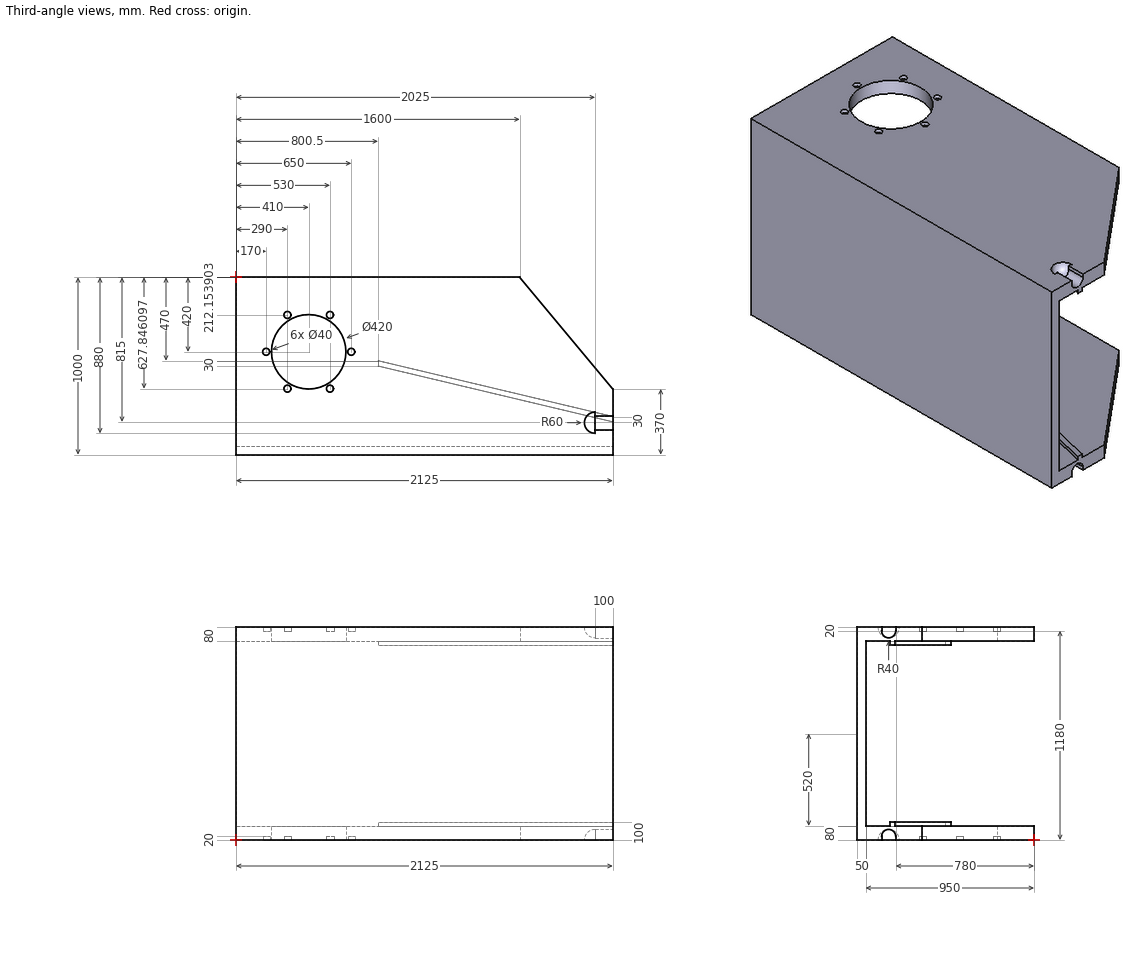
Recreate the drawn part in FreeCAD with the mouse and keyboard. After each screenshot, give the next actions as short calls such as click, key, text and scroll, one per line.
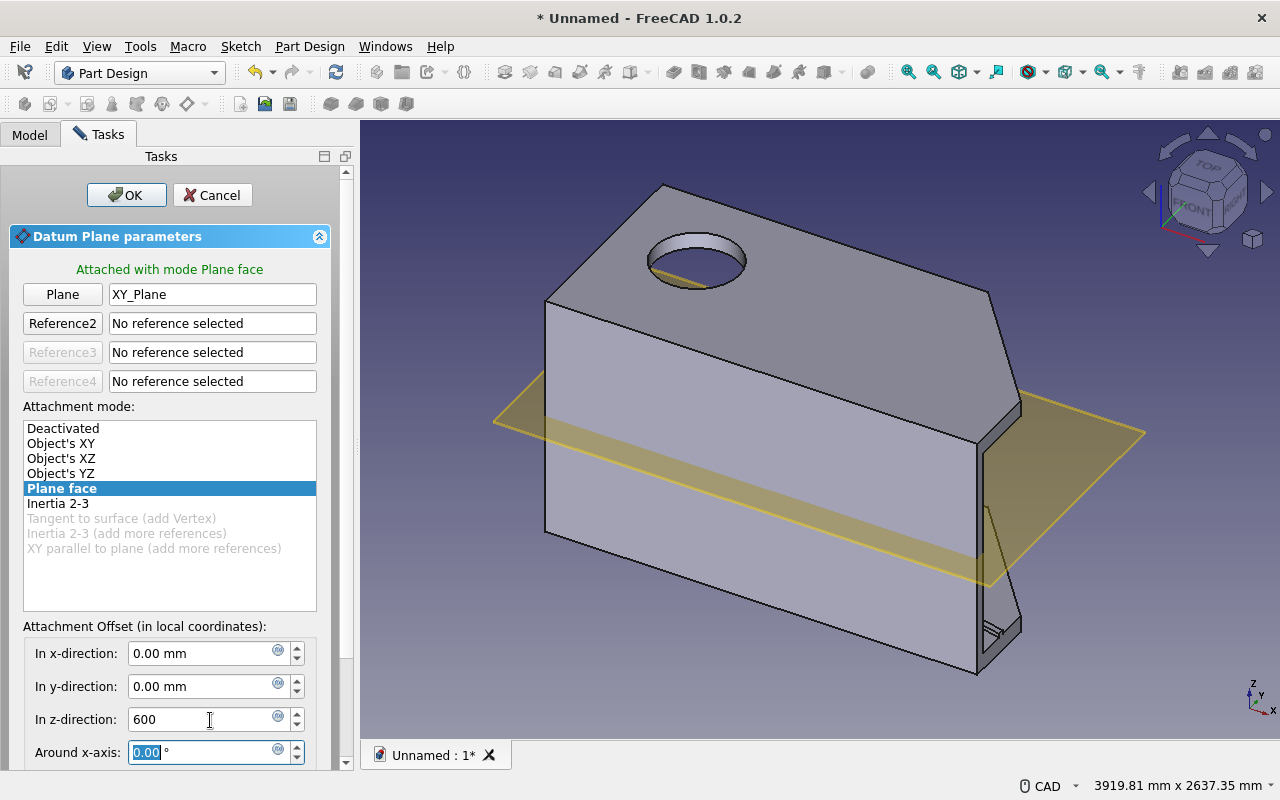
click(127, 195)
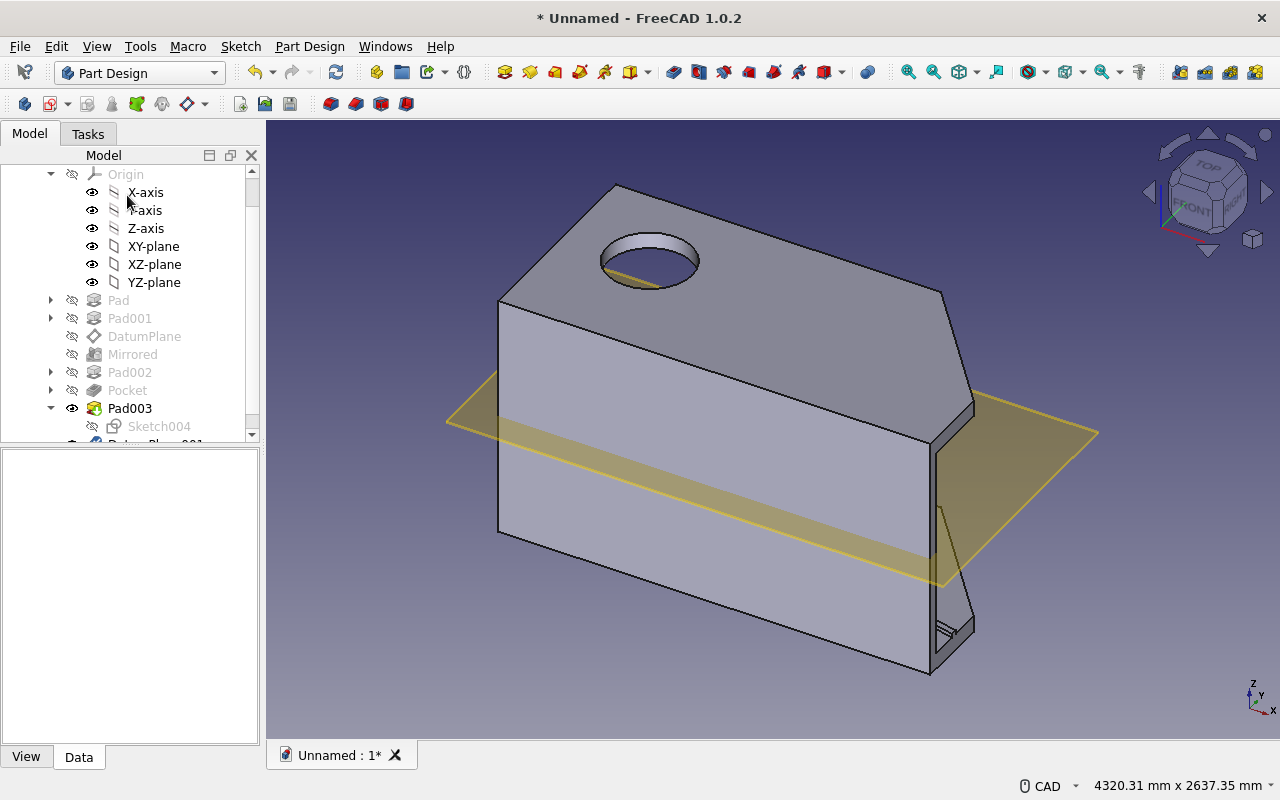
click(117, 408)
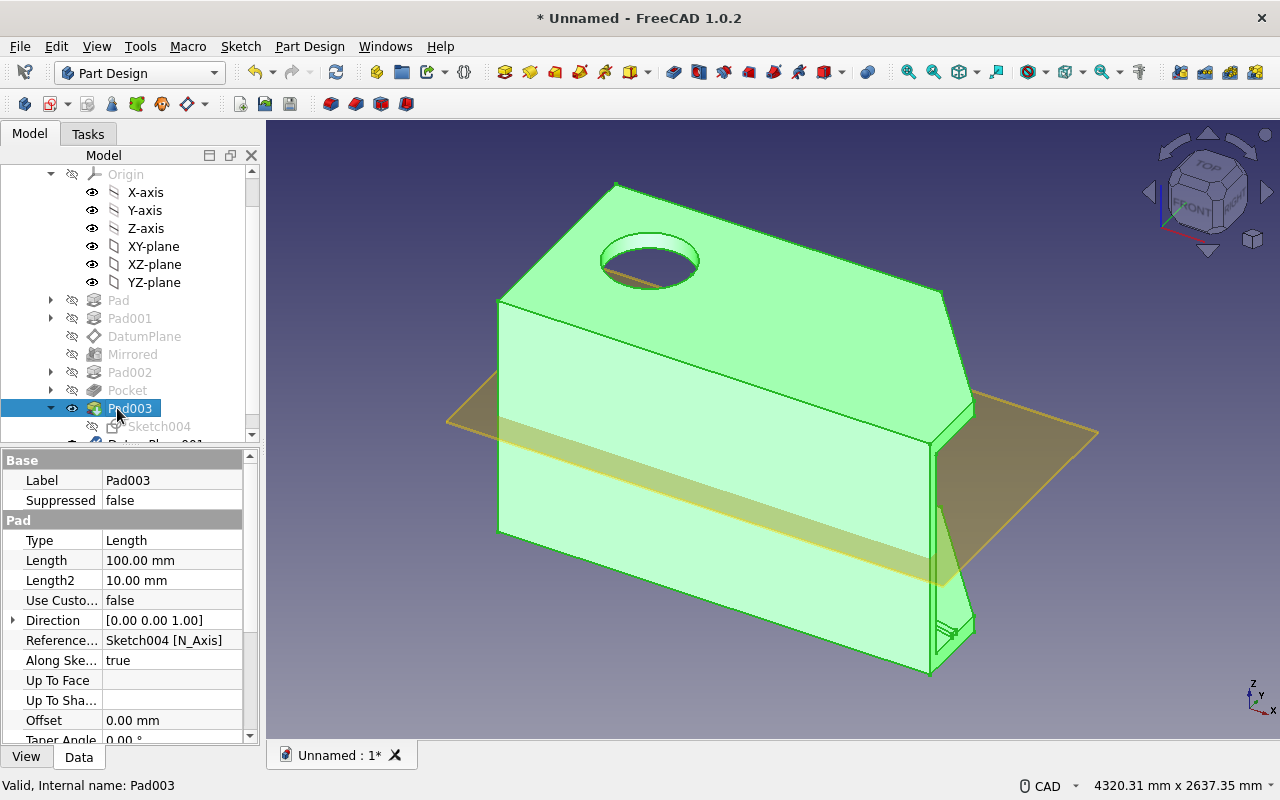
click(1180, 72)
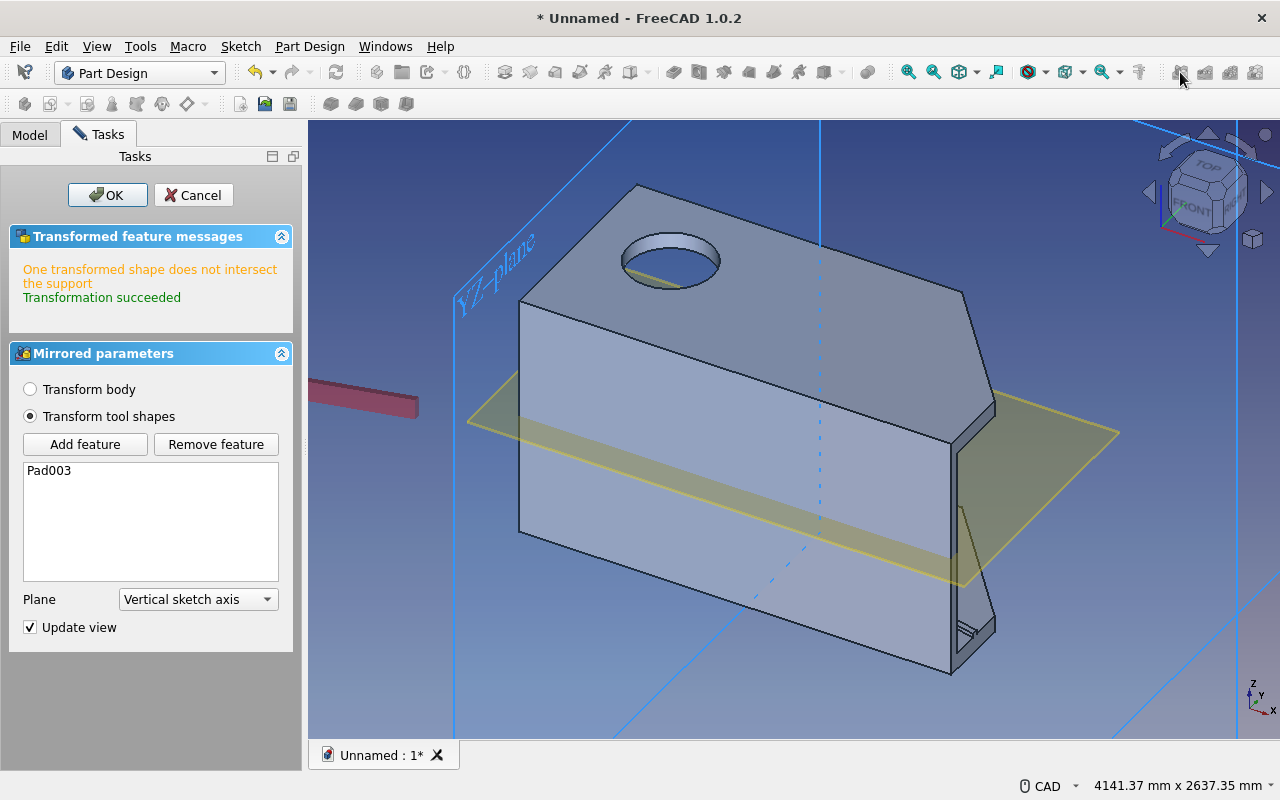
click(199, 600)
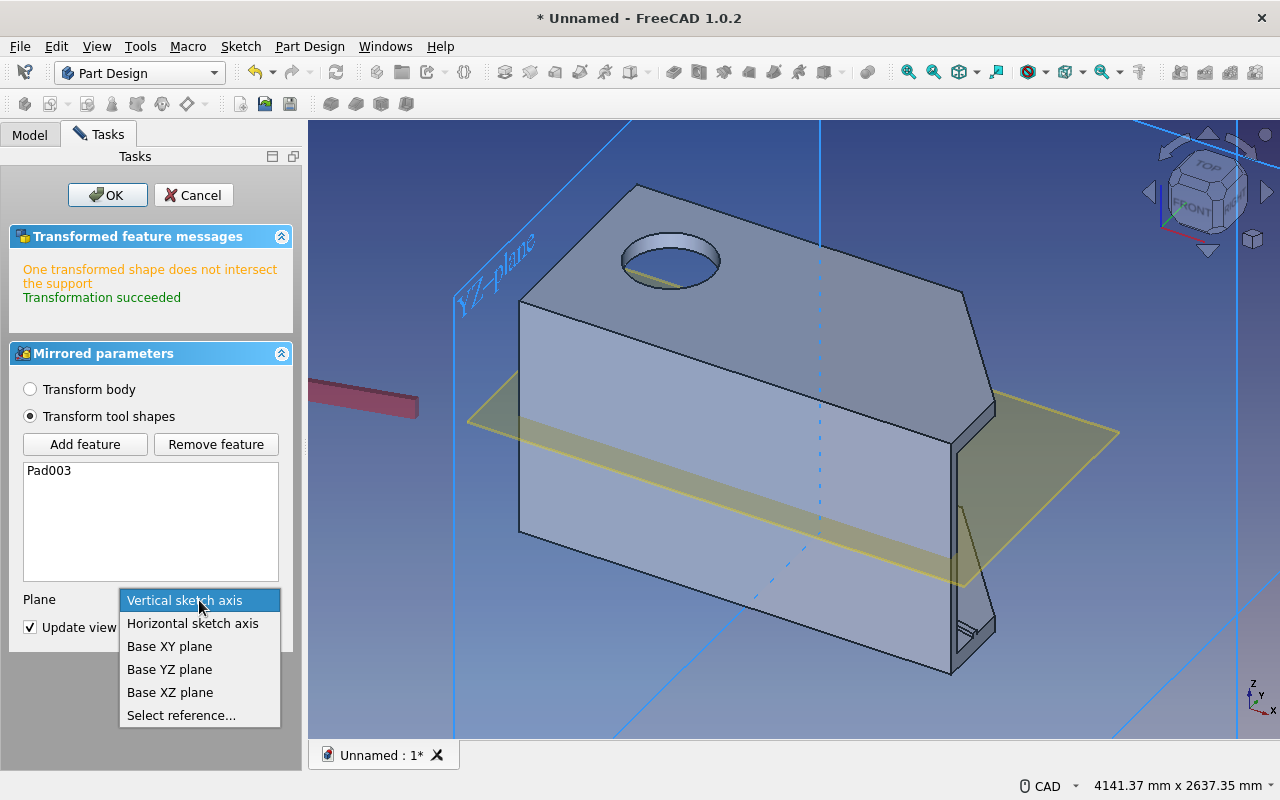
click(198, 716)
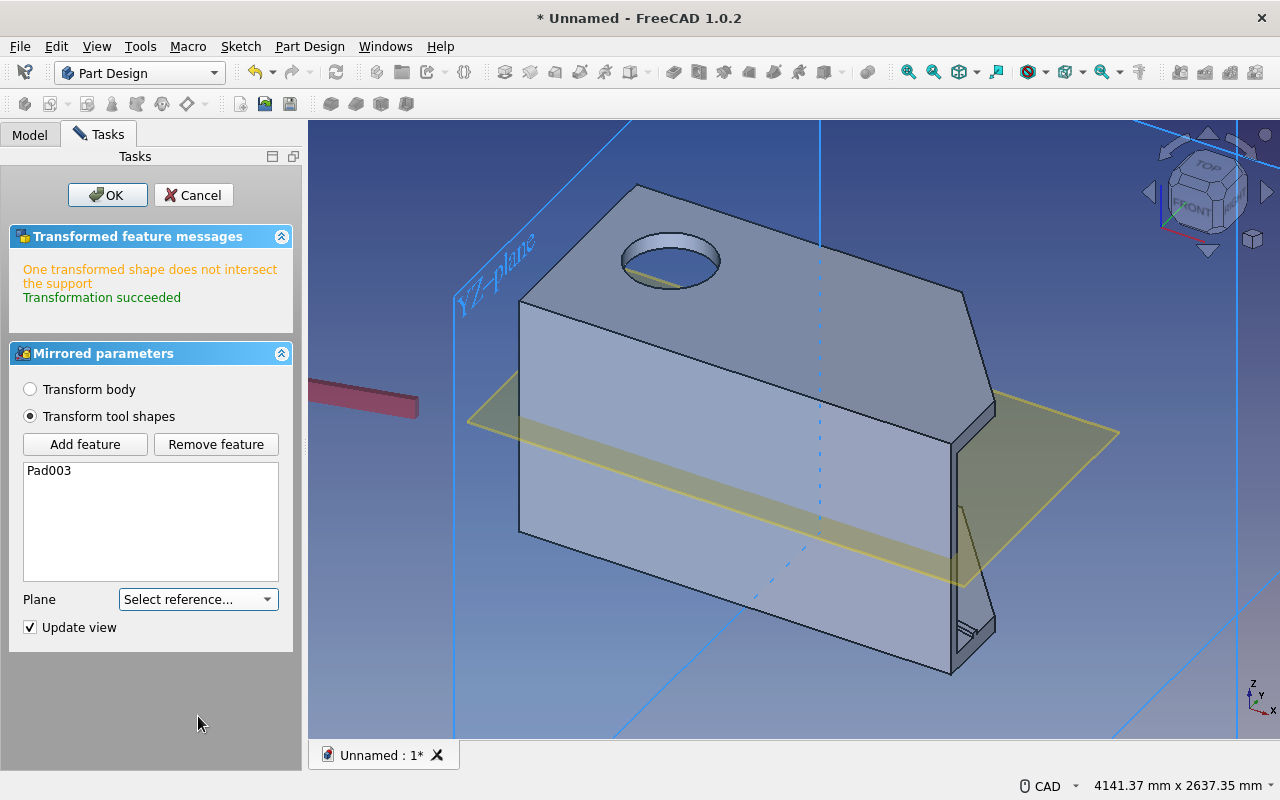
click(30, 134)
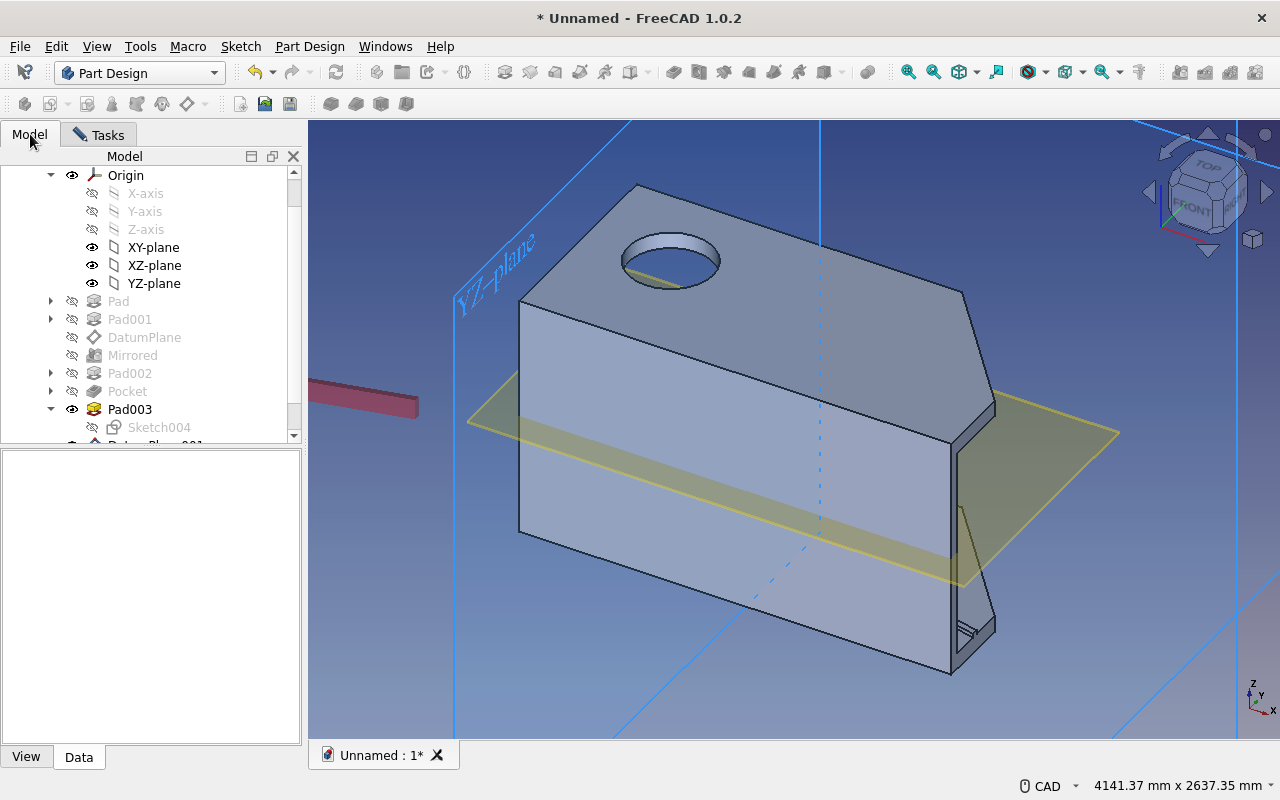
scroll(141, 297, down, 3)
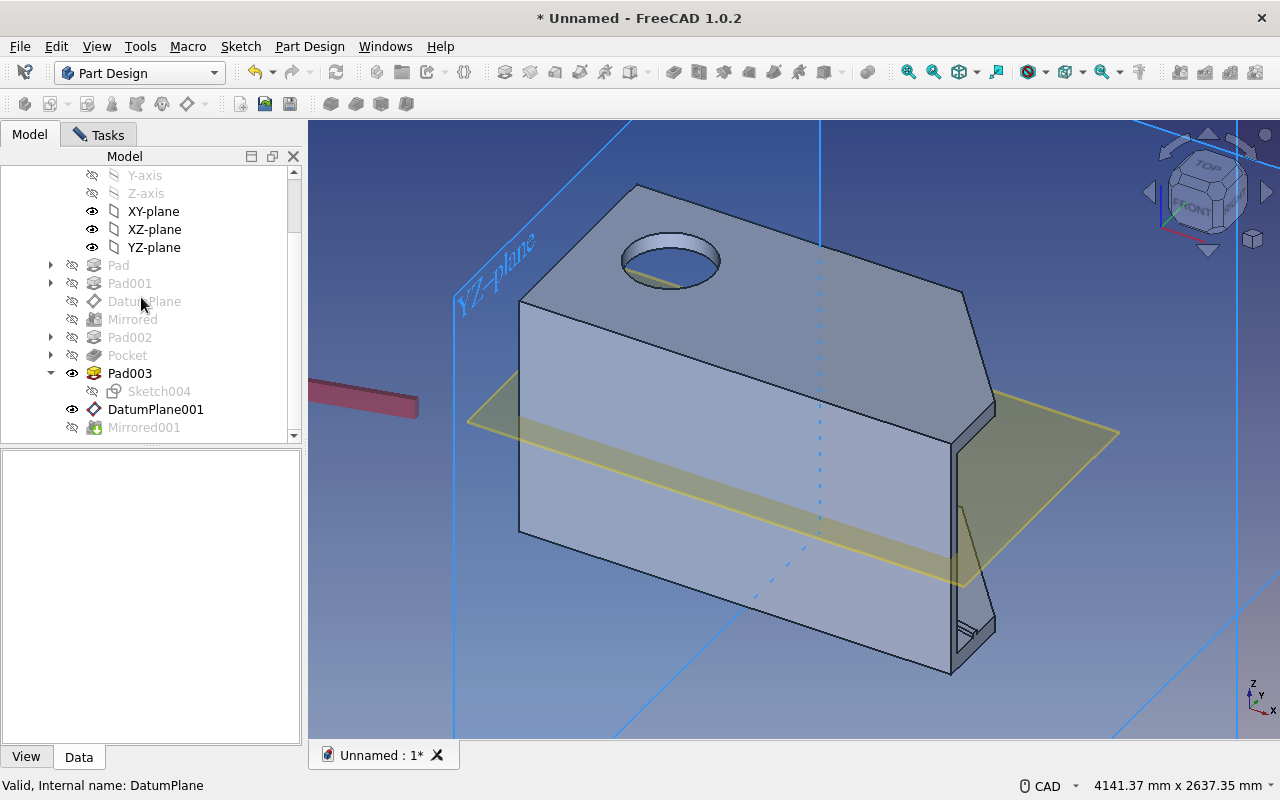
click(117, 409)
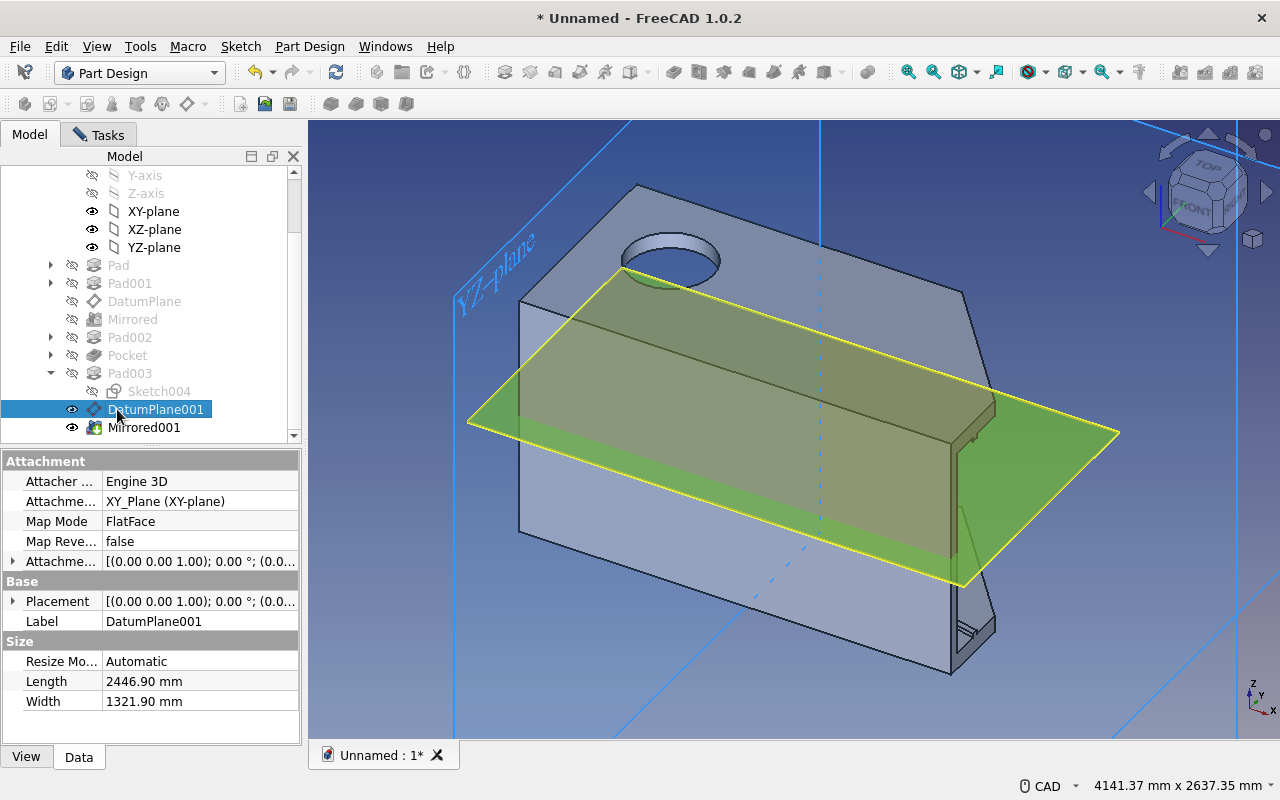
click(98, 134)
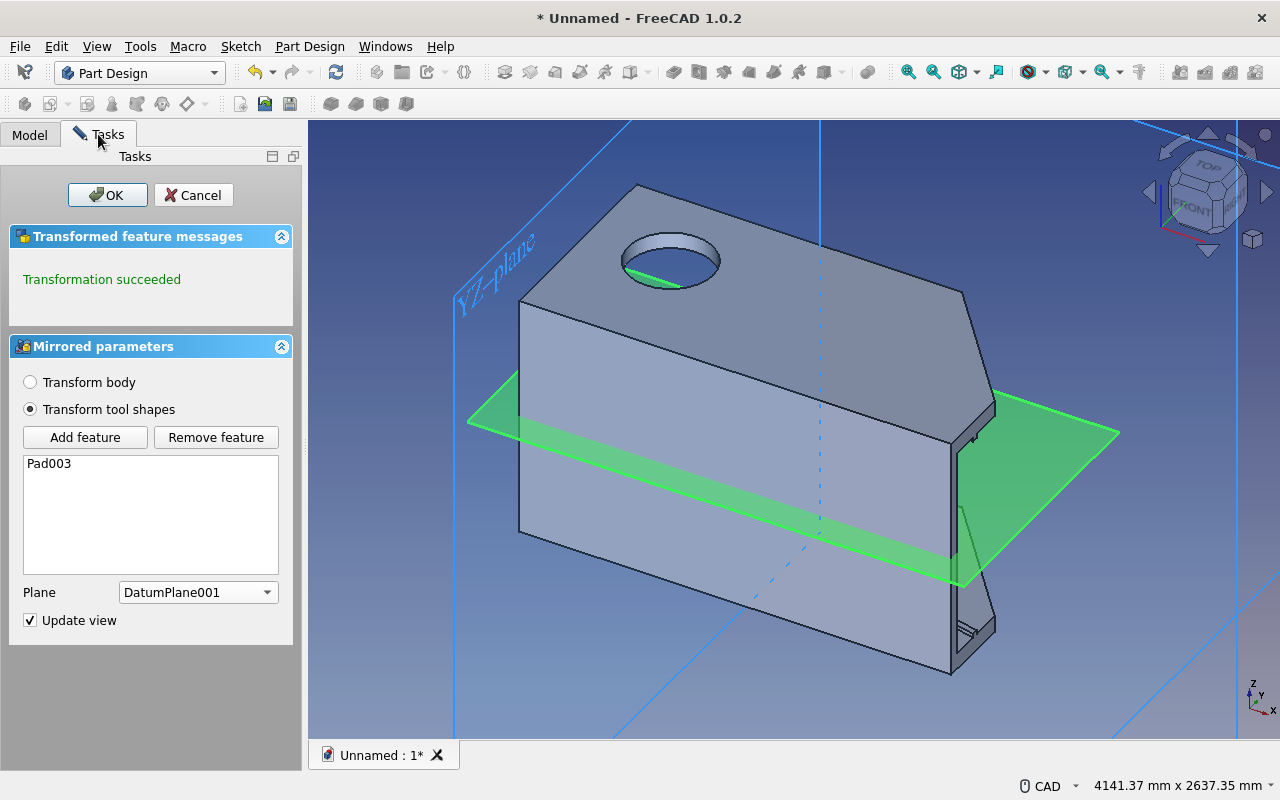
click(108, 195)